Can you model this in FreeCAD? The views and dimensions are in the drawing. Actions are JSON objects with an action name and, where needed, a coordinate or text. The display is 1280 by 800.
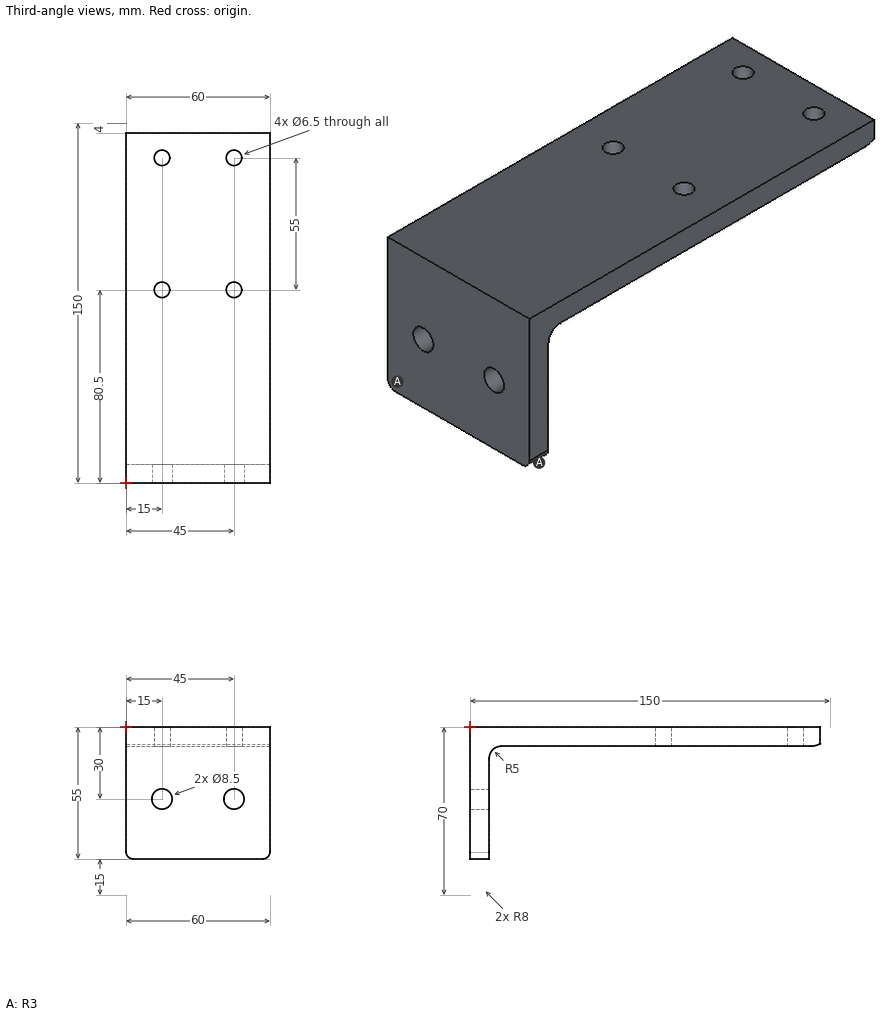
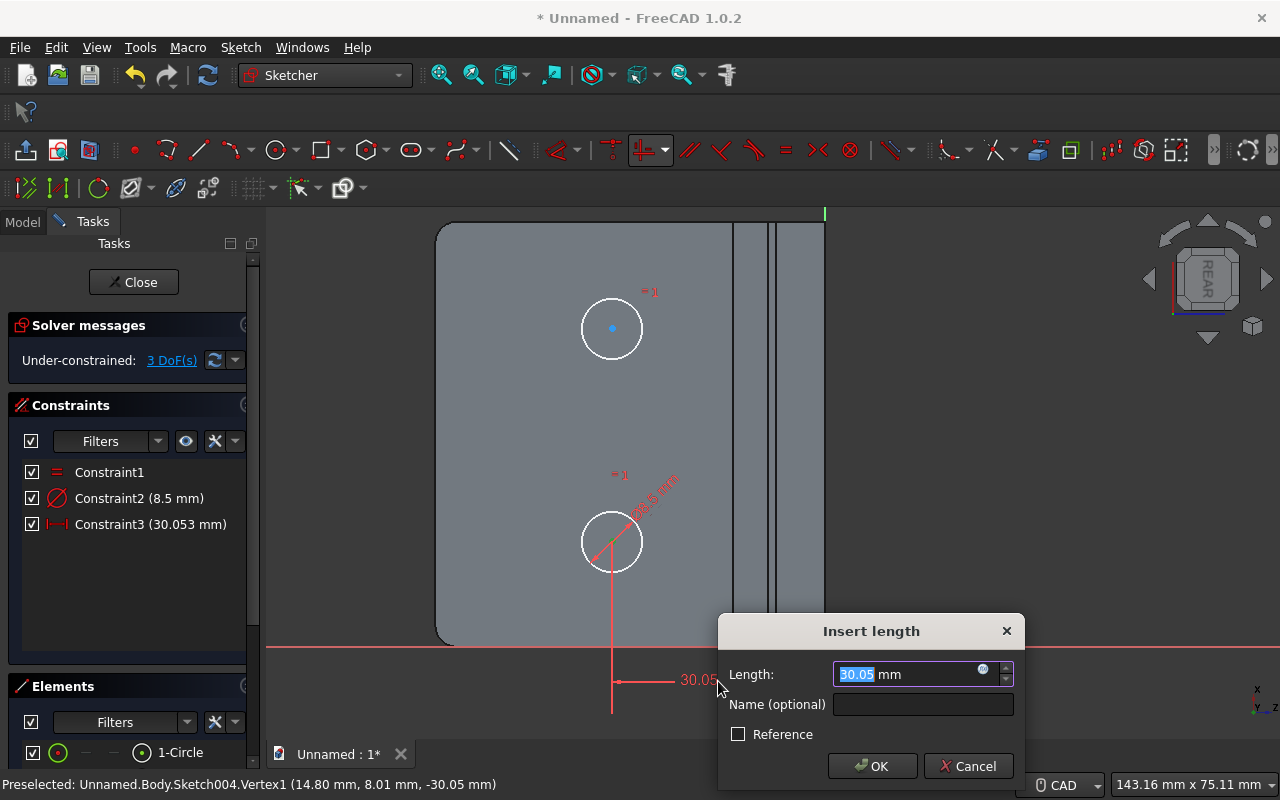
{"action": "type", "text": "30"}
{"action": "key", "text": "Return"}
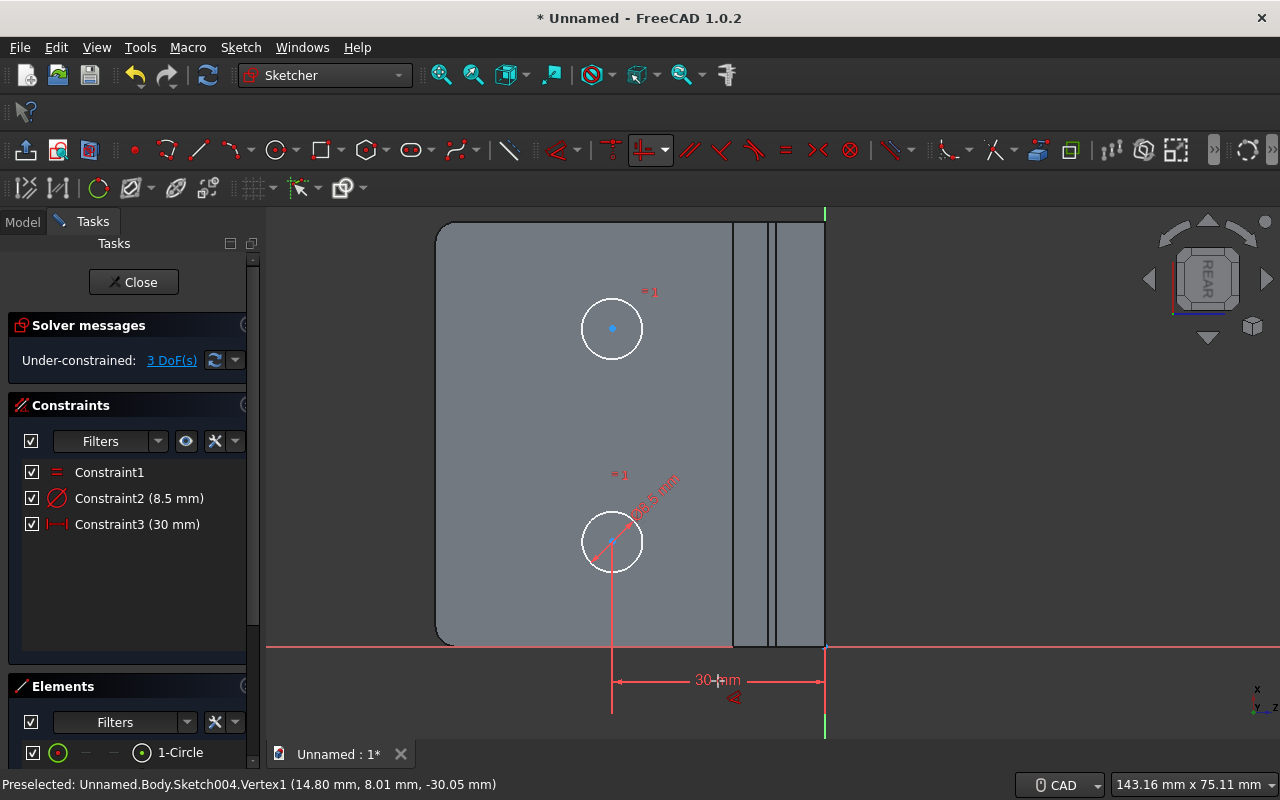
{"action": "left_click", "coordinate": [612, 542]}
{"action": "left_click", "coordinate": [859, 594]}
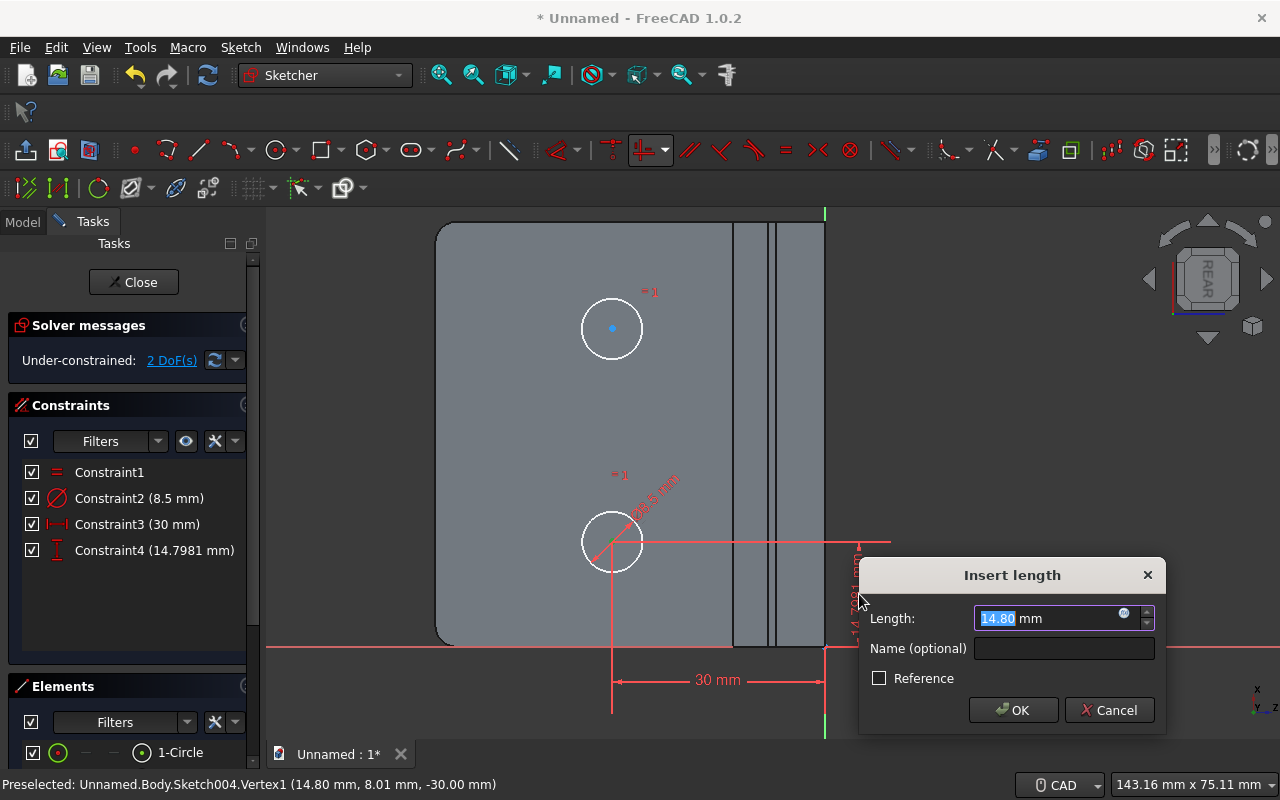
{"action": "type", "text": "15"}
{"action": "key", "text": "Return"}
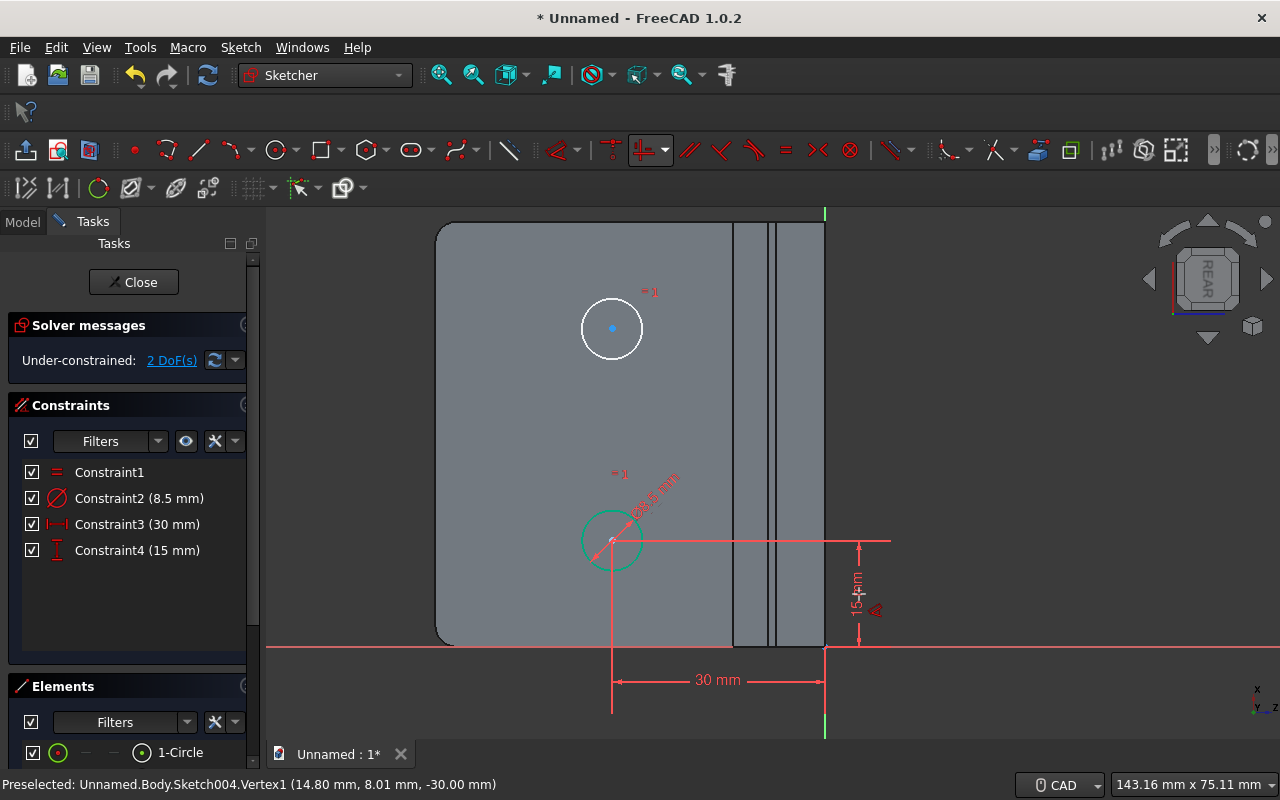
{"action": "left_click", "coordinate": [612, 329]}
{"action": "left_click", "coordinate": [644, 681]}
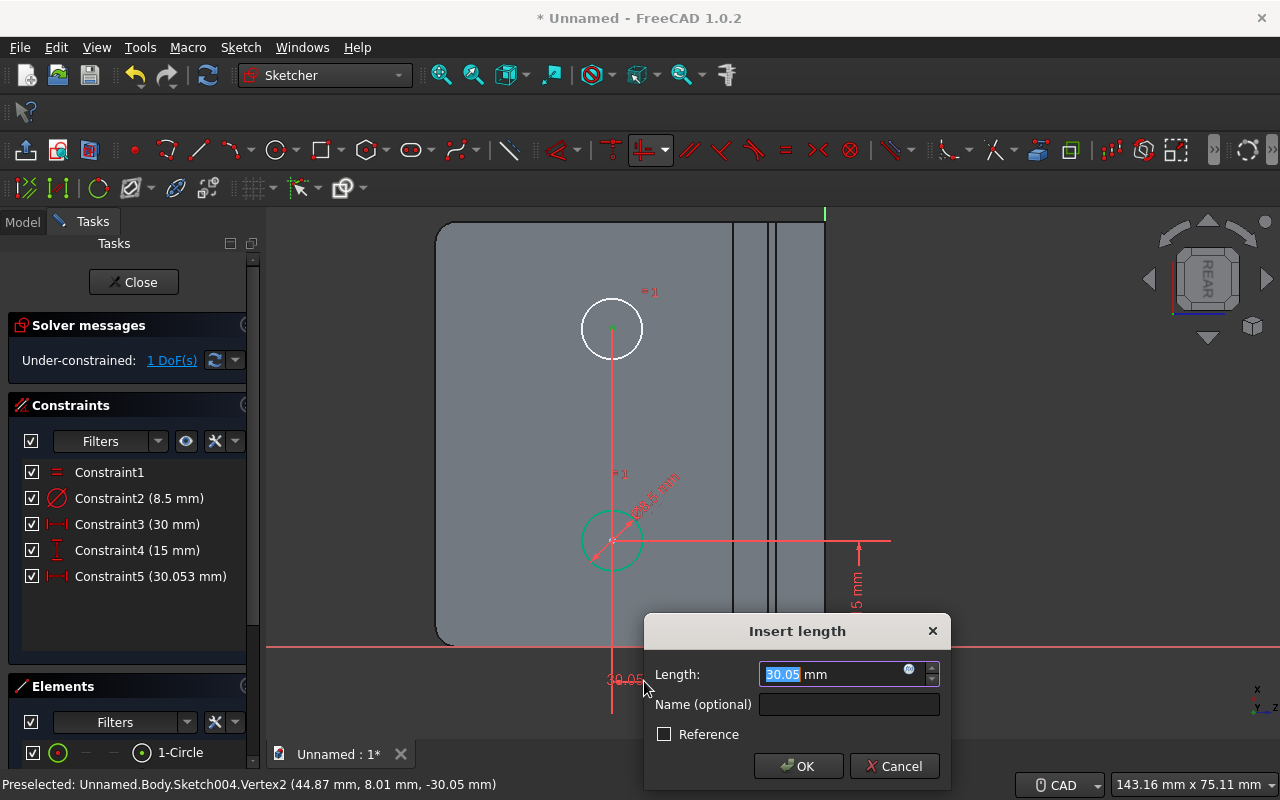
{"action": "type", "text": "30"}
{"action": "key", "text": "Return"}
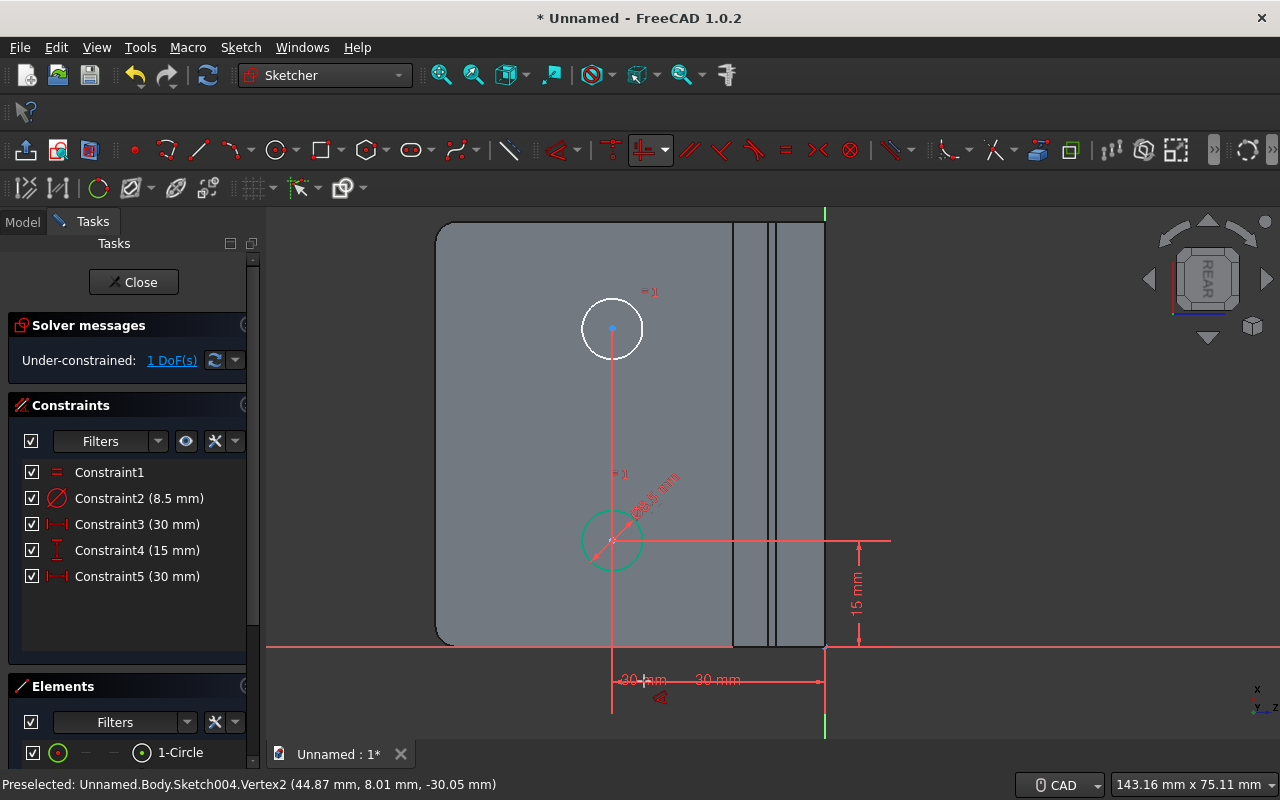
{"action": "left_click", "coordinate": [612, 329]}
{"action": "left_click", "coordinate": [859, 488]}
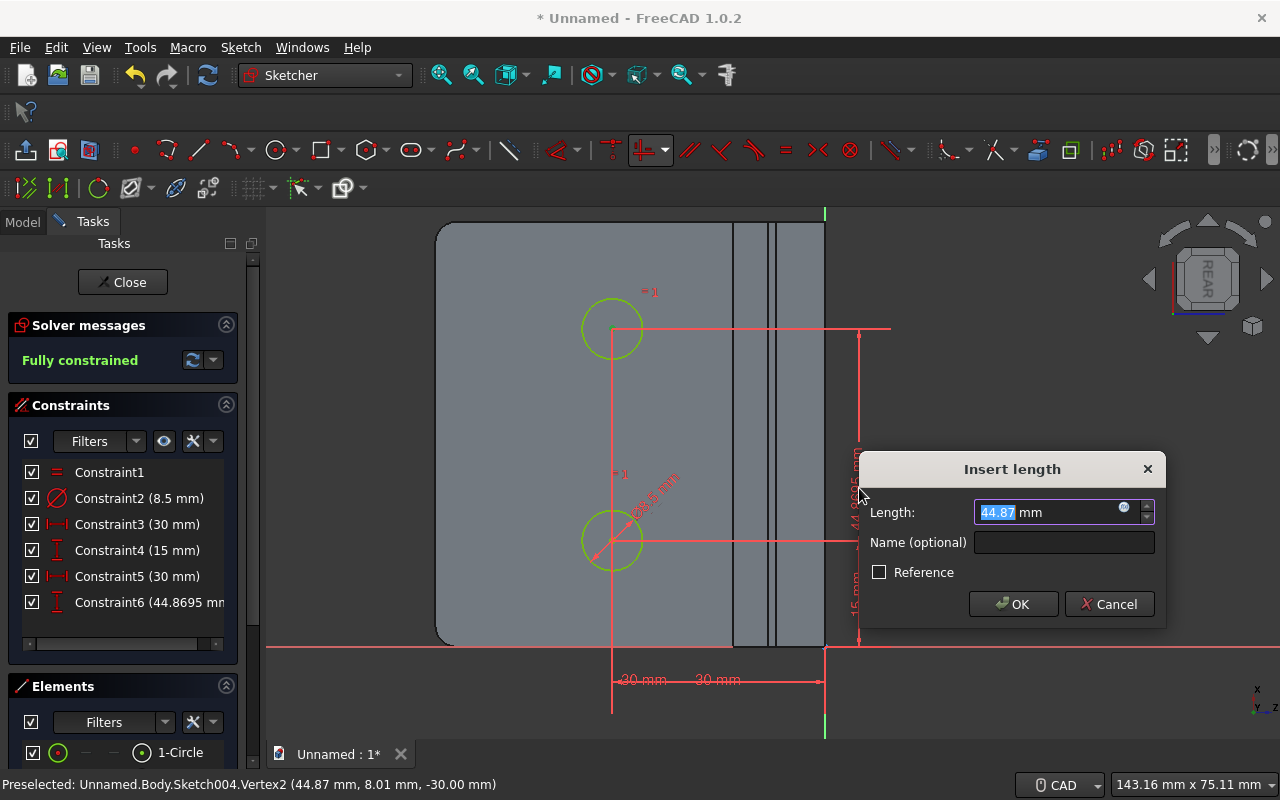
{"action": "type", "text": "45"}
{"action": "key", "text": "Return"}
{"action": "key", "text": "Escape"}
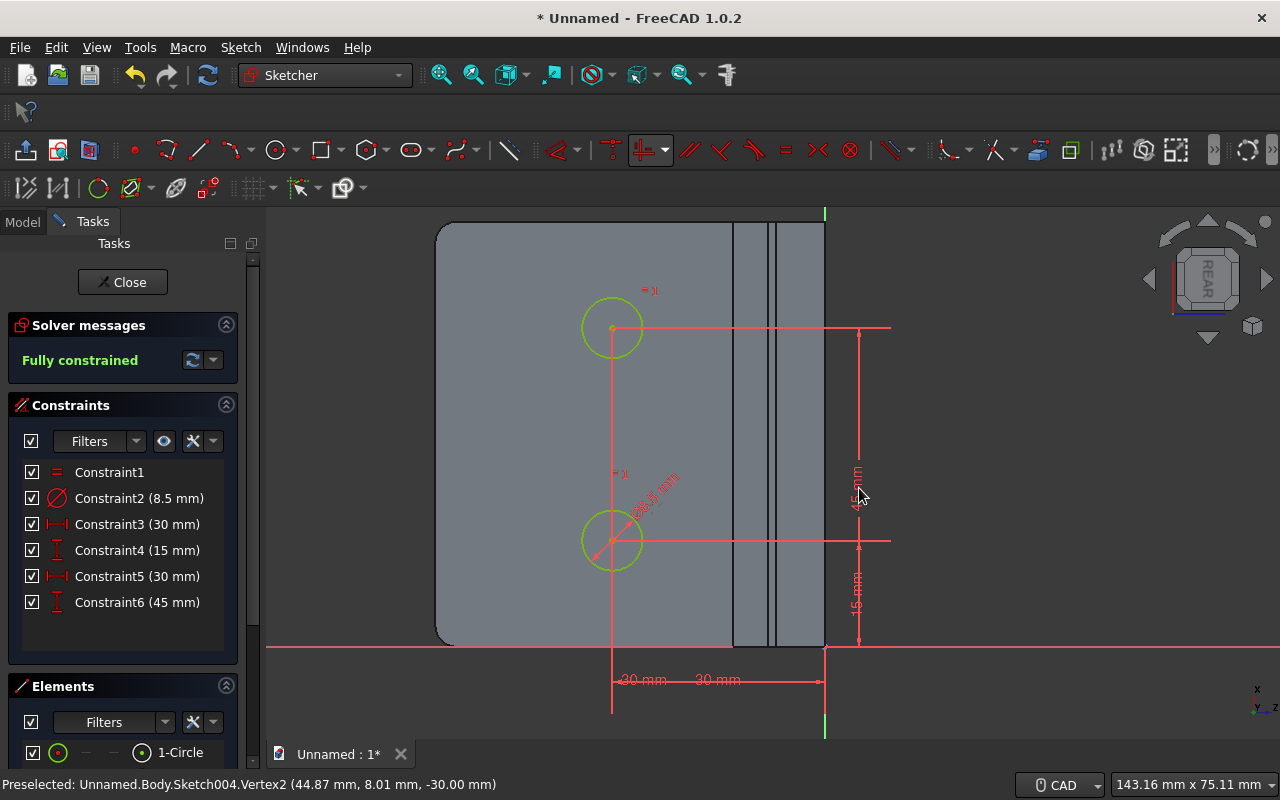
{"action": "left_click", "coordinate": [123, 282]}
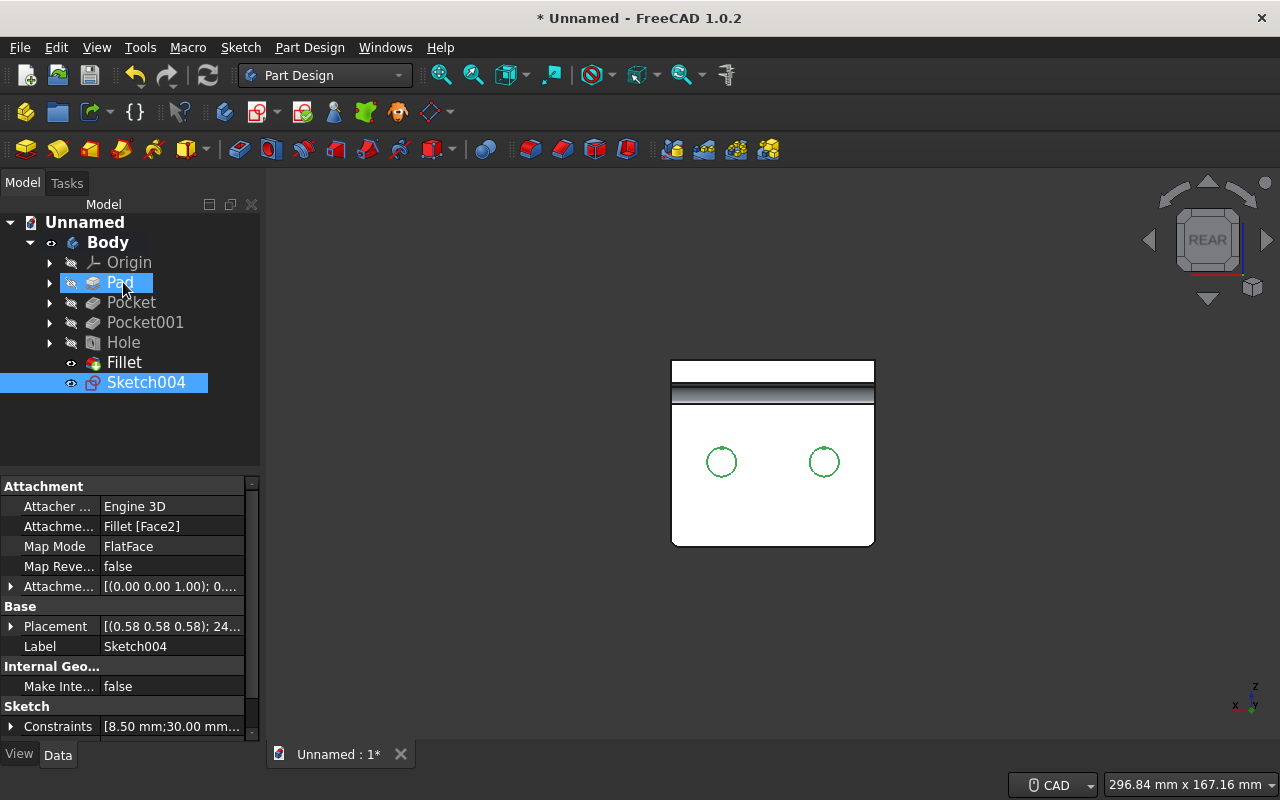
{"action": "left_click", "coordinate": [240, 150]}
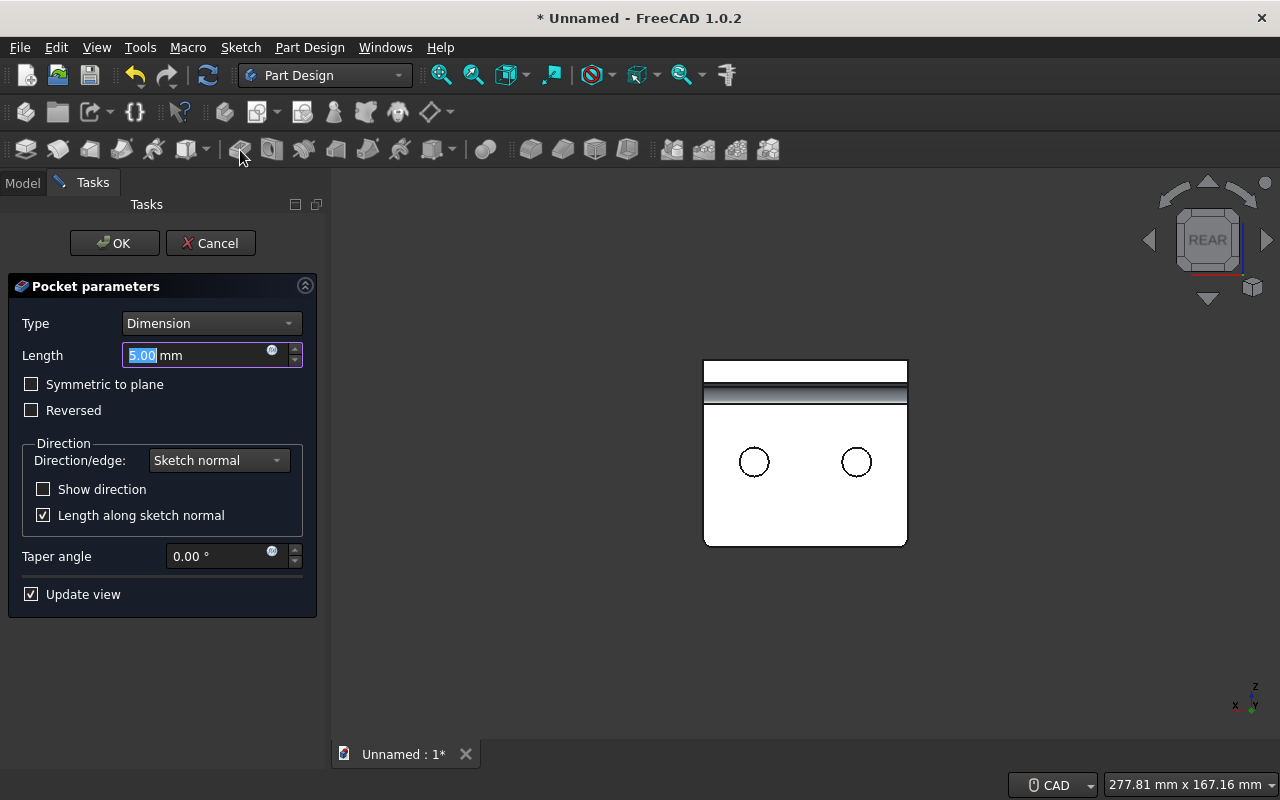
{"action": "left_click", "coordinate": [212, 324]}